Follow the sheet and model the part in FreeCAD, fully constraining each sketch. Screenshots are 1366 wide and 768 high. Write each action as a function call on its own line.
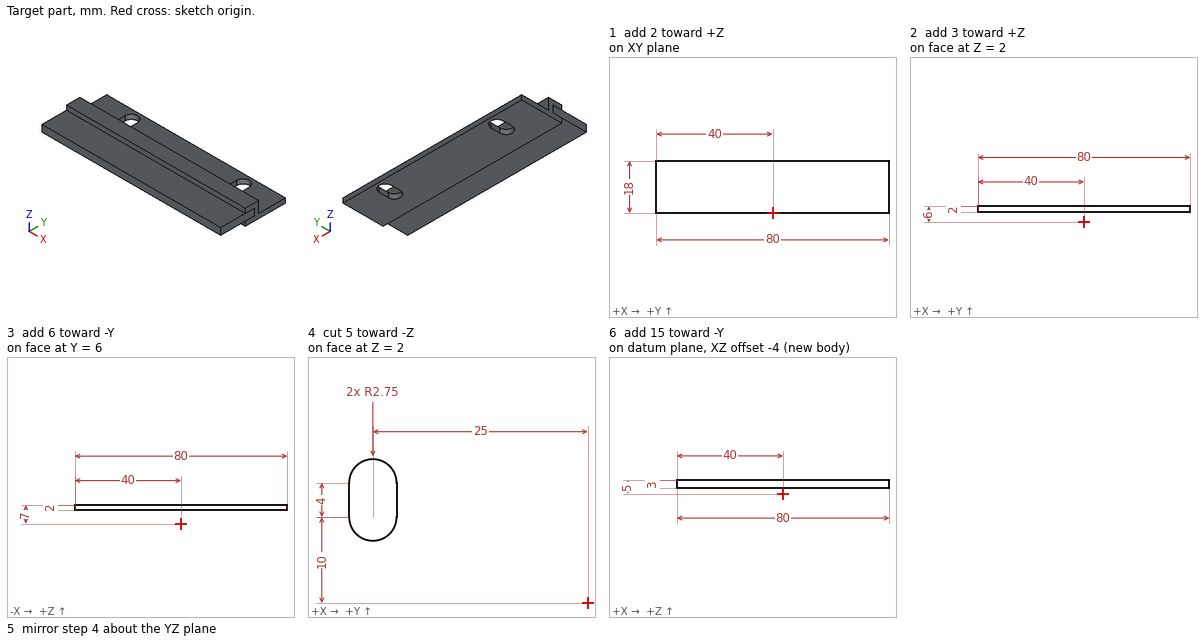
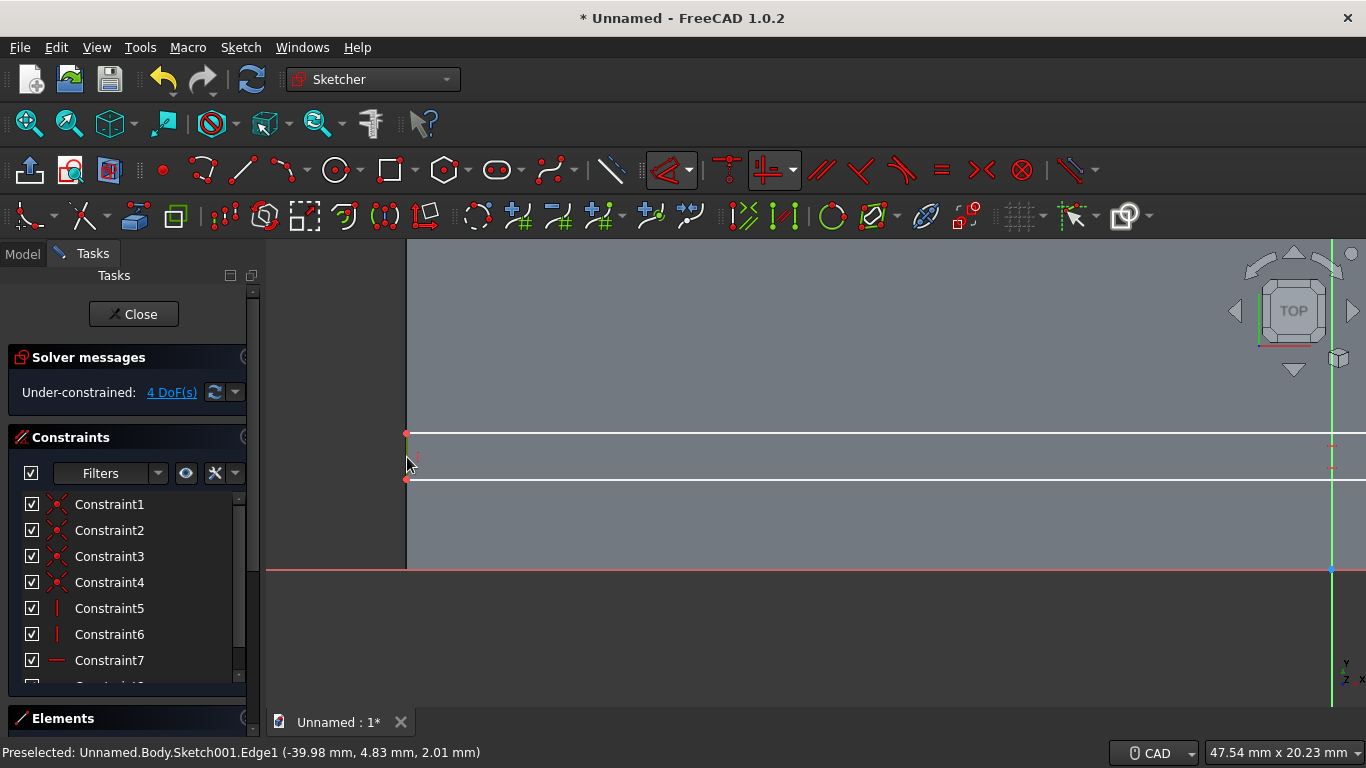
click(692, 170)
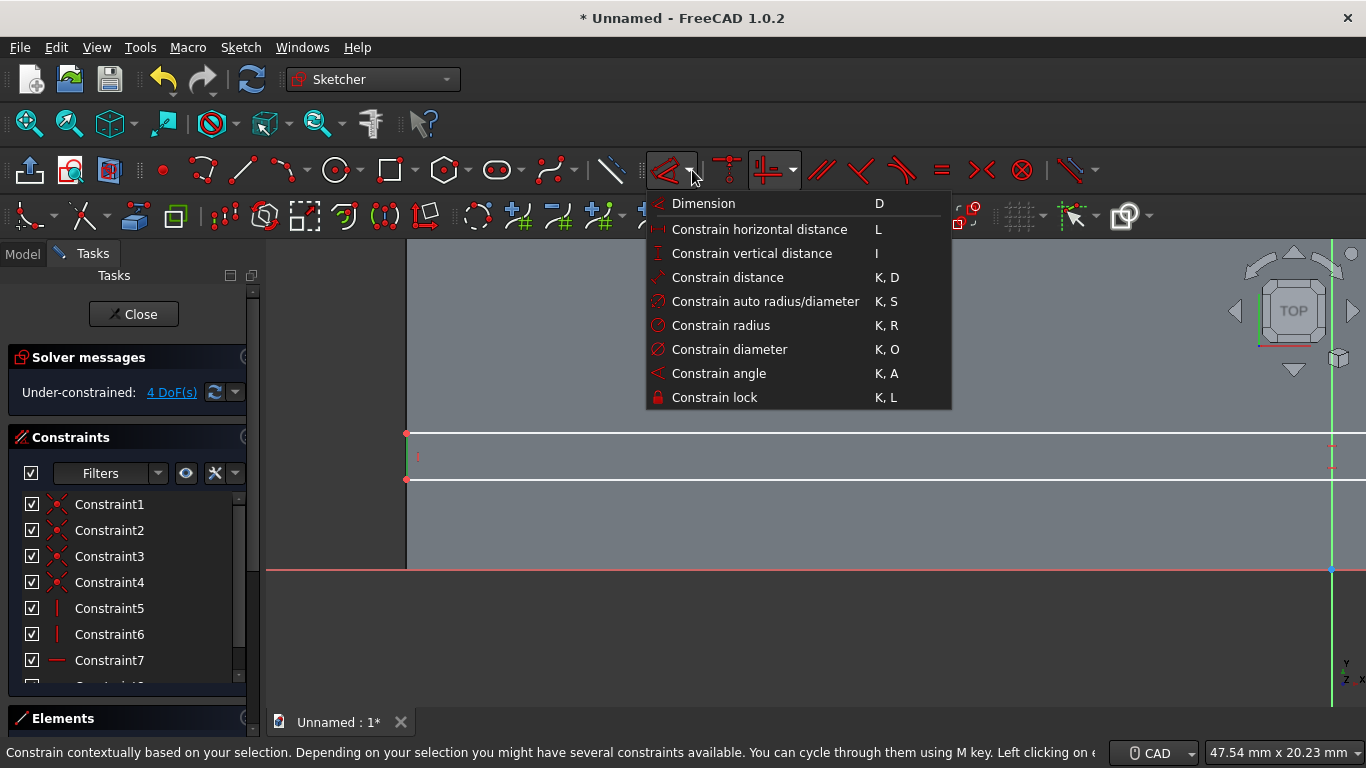
click(799, 253)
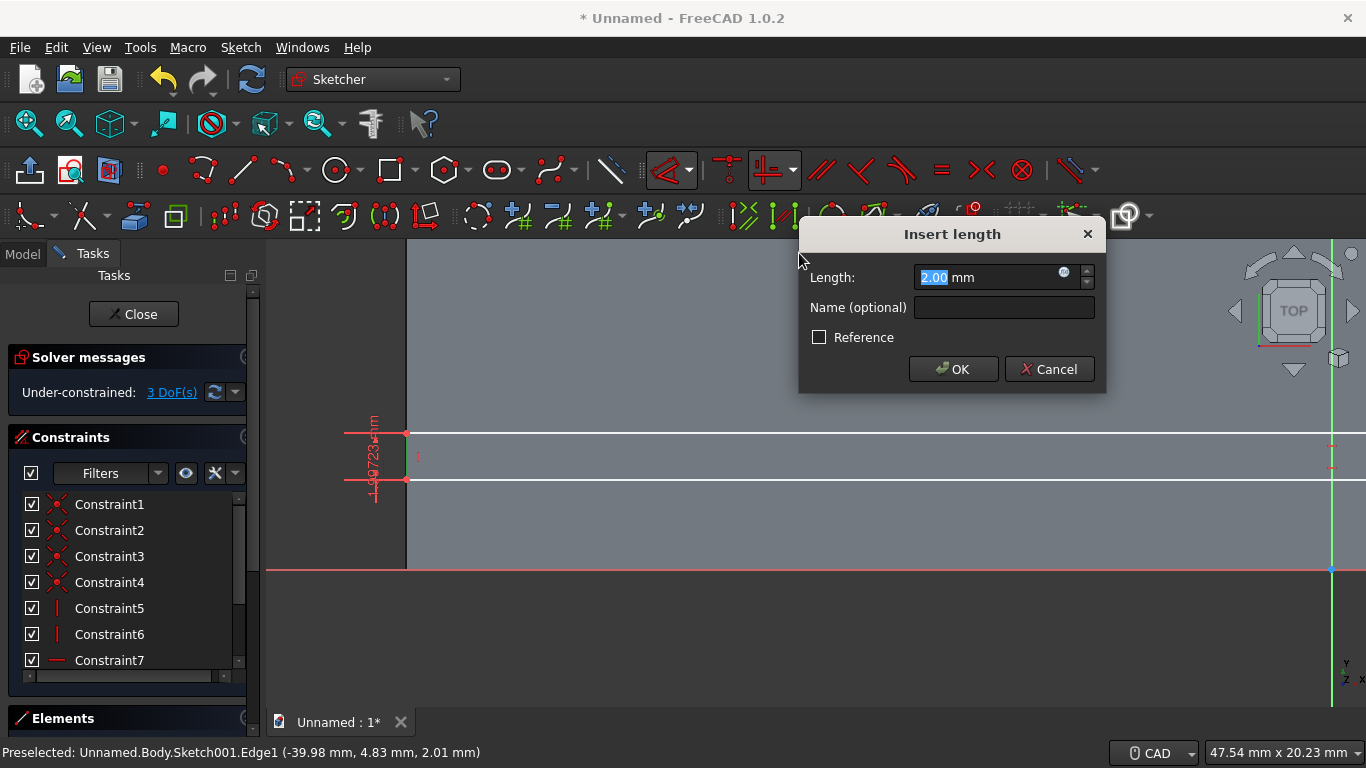
text(2)
key(Return)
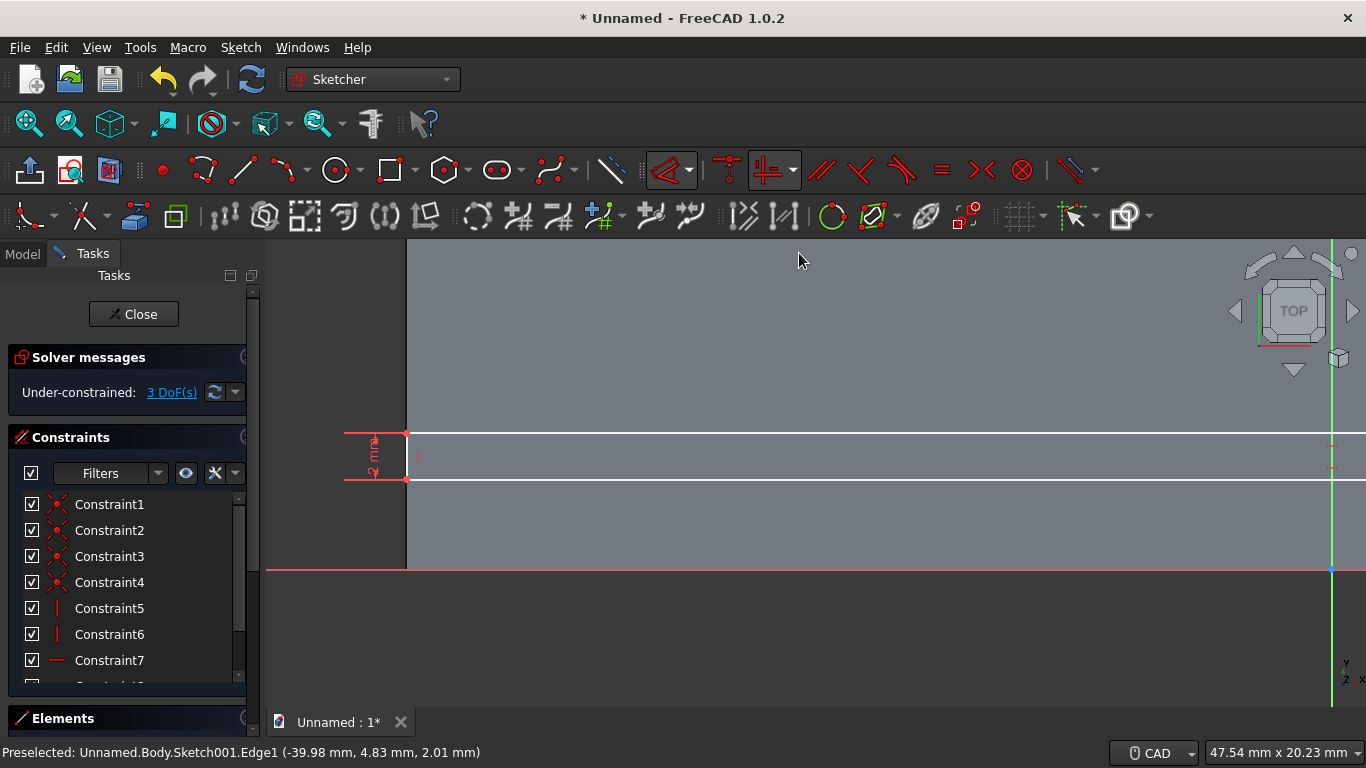
click(962, 480)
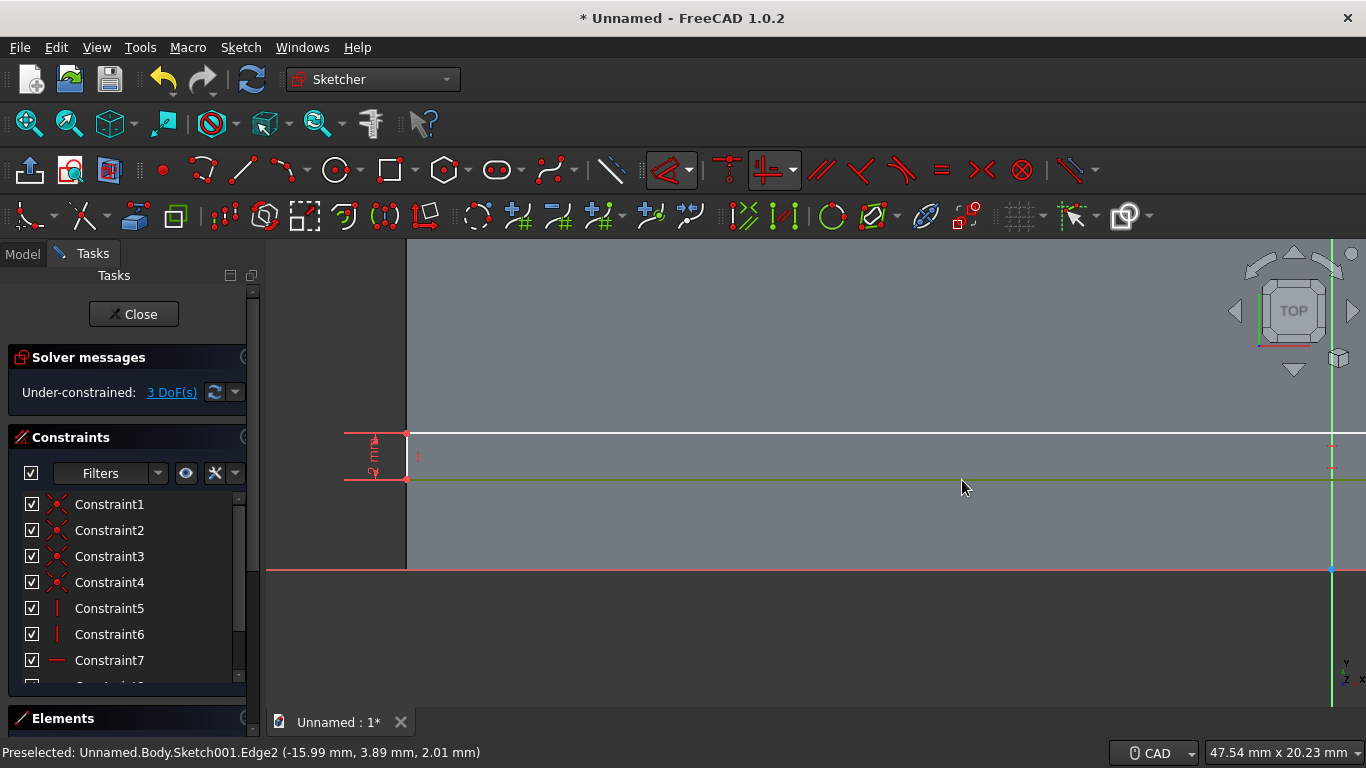
click(692, 170)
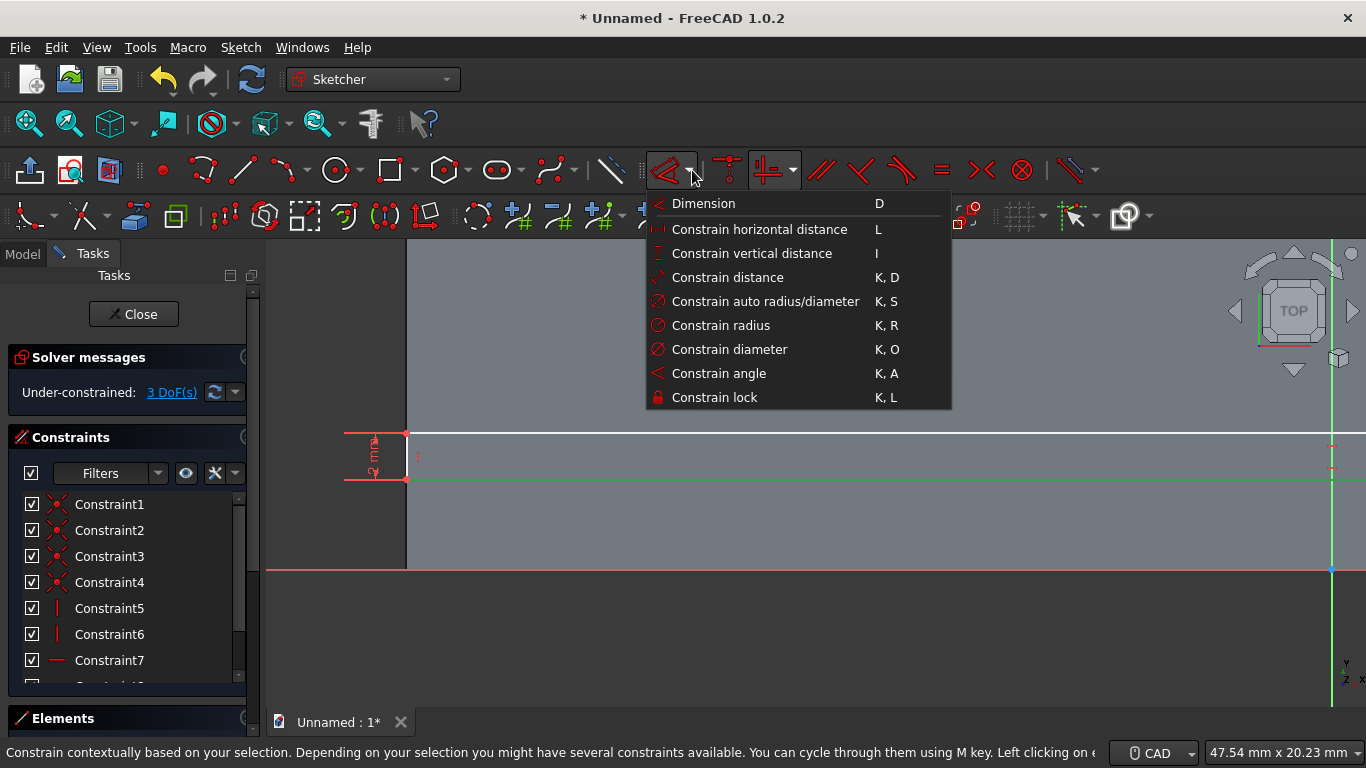
click(799, 229)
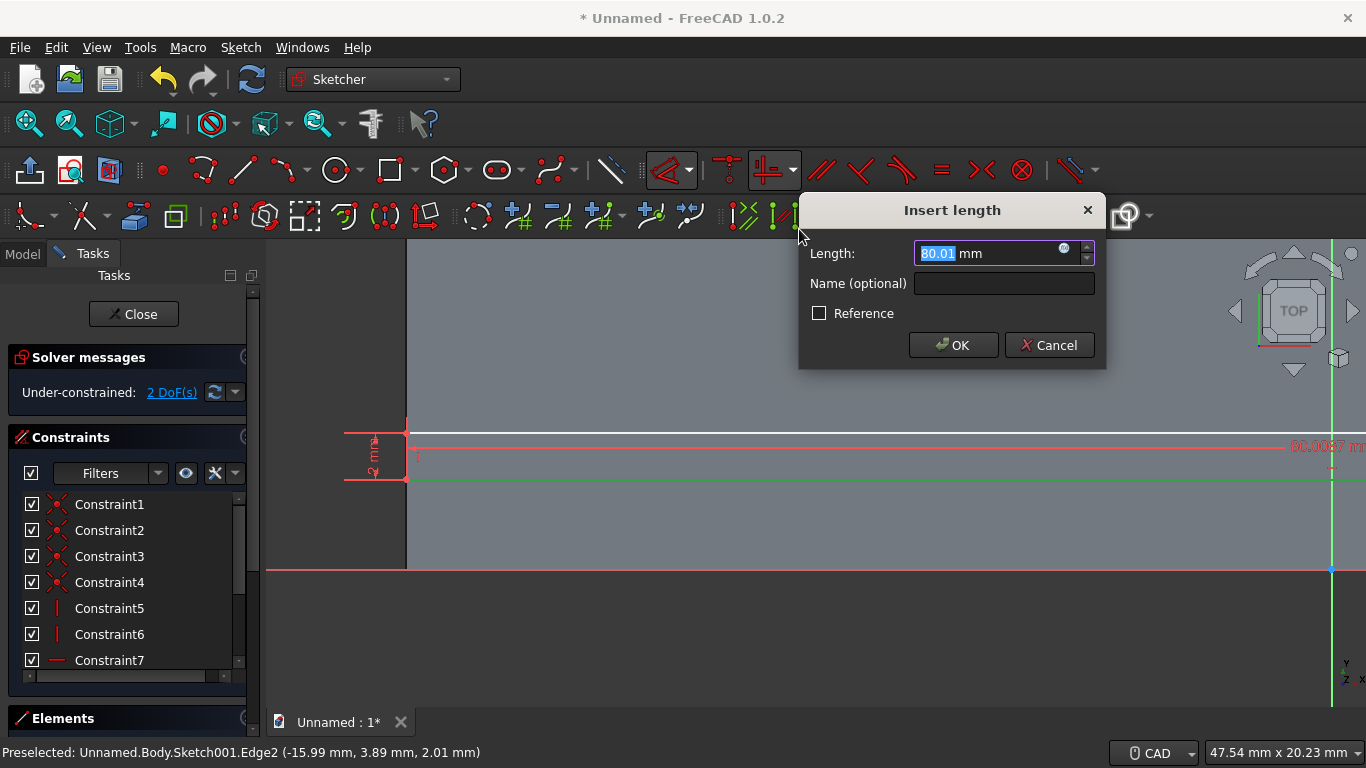
text(80)
key(Return)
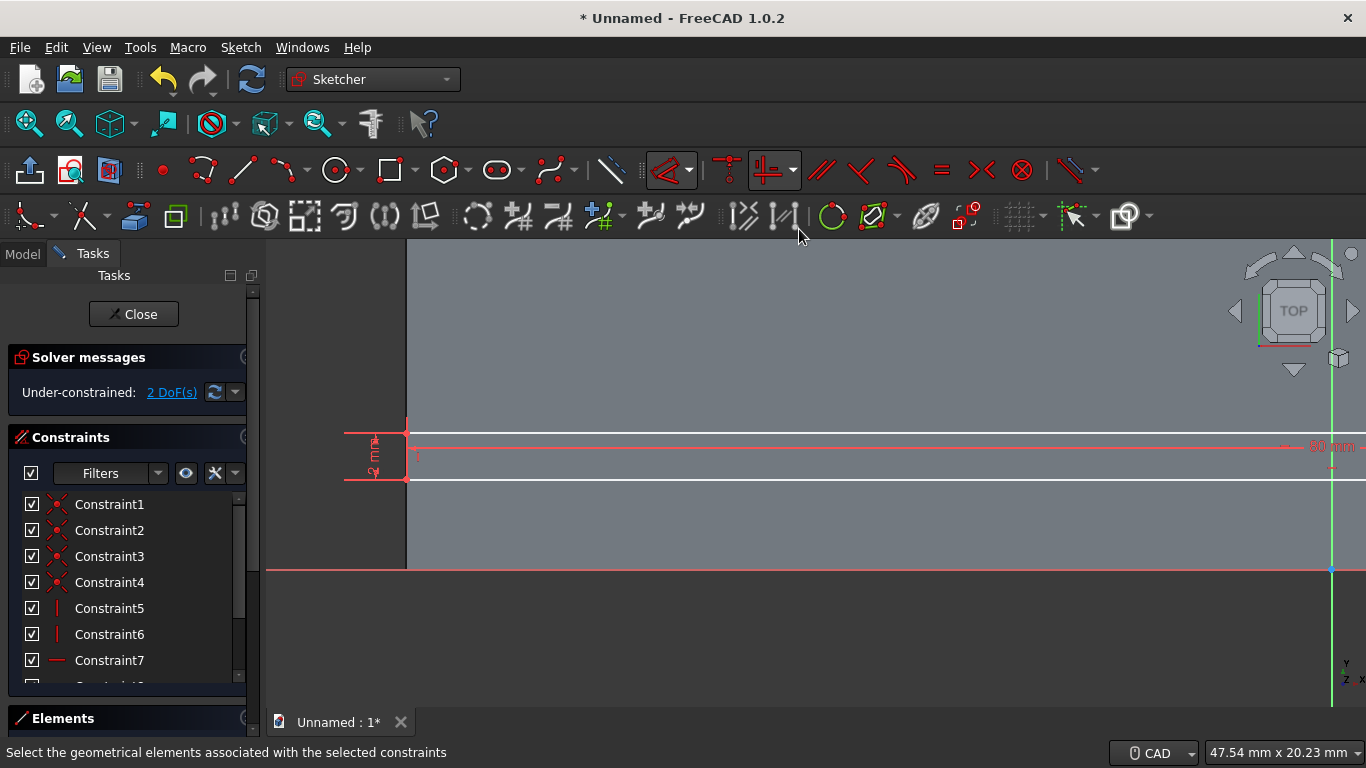
click(407, 433)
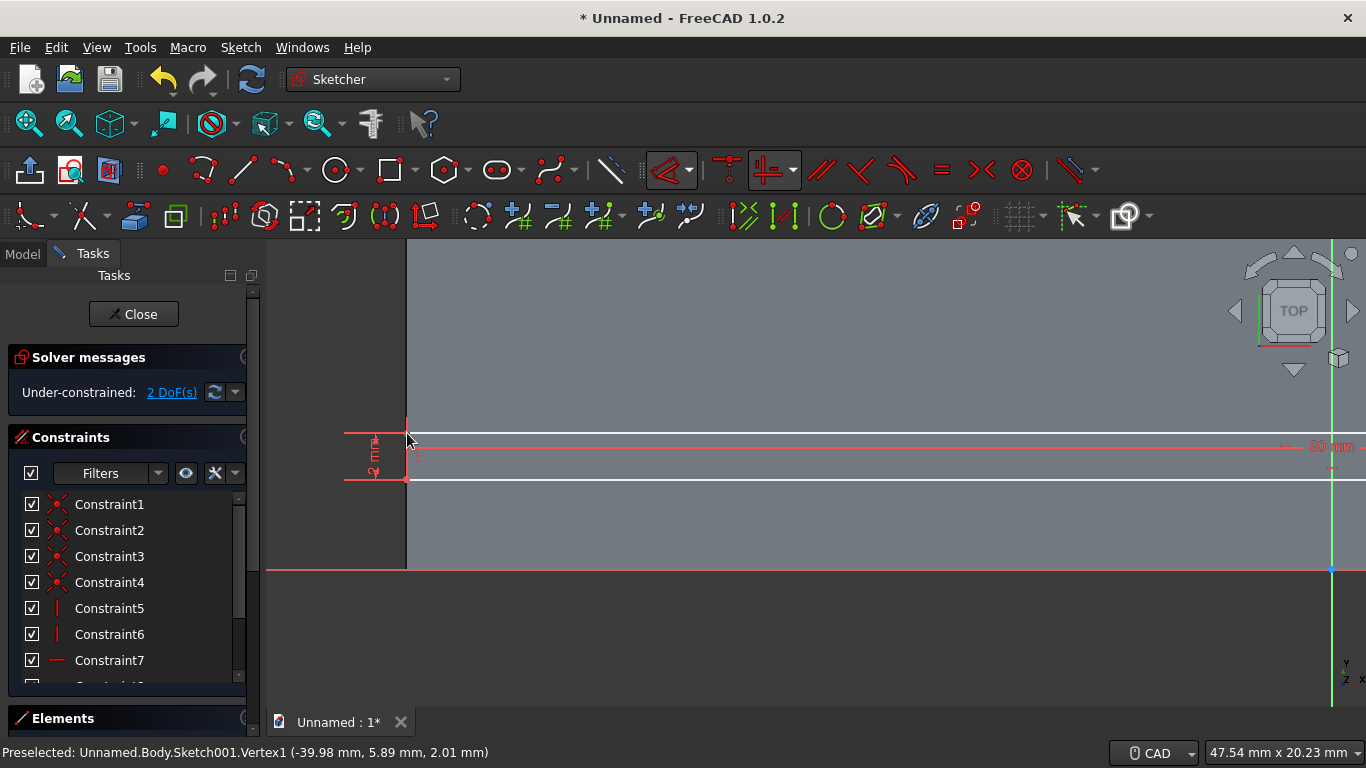
click(692, 170)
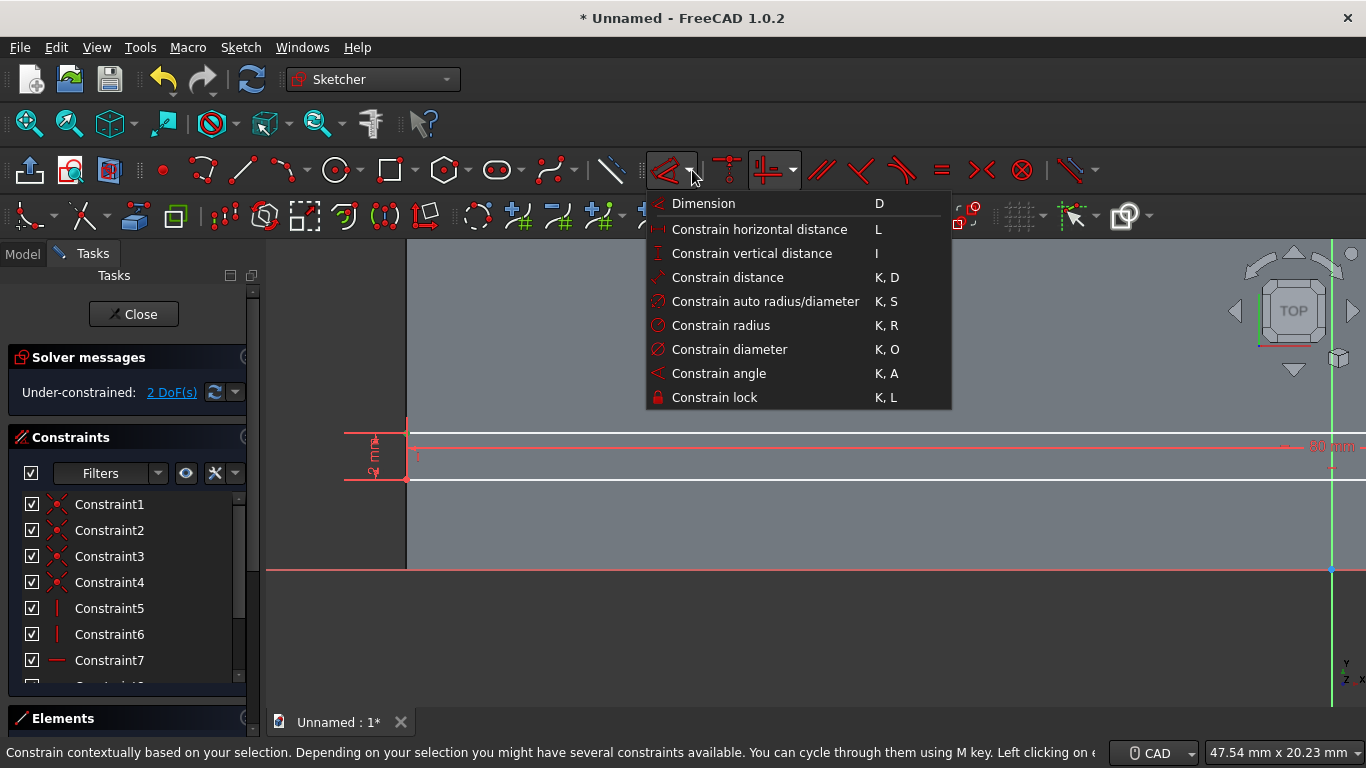
click(799, 253)